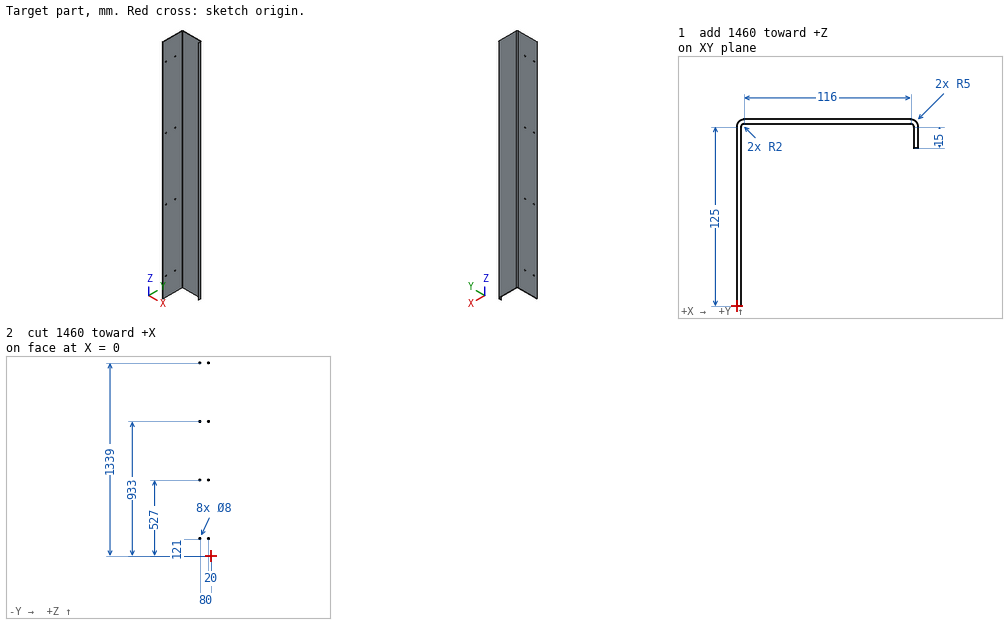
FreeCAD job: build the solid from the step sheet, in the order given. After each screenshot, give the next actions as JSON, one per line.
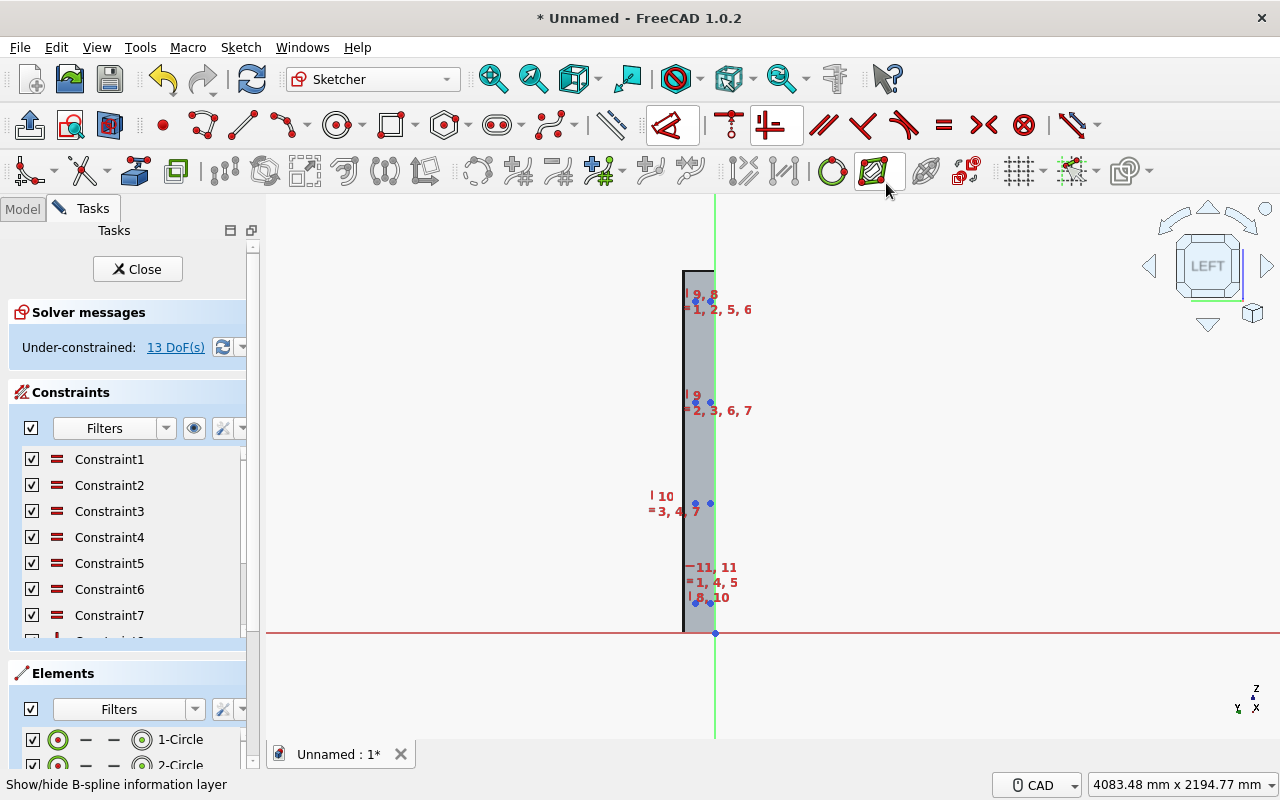
{"action": "left_click", "coordinate": [710, 604]}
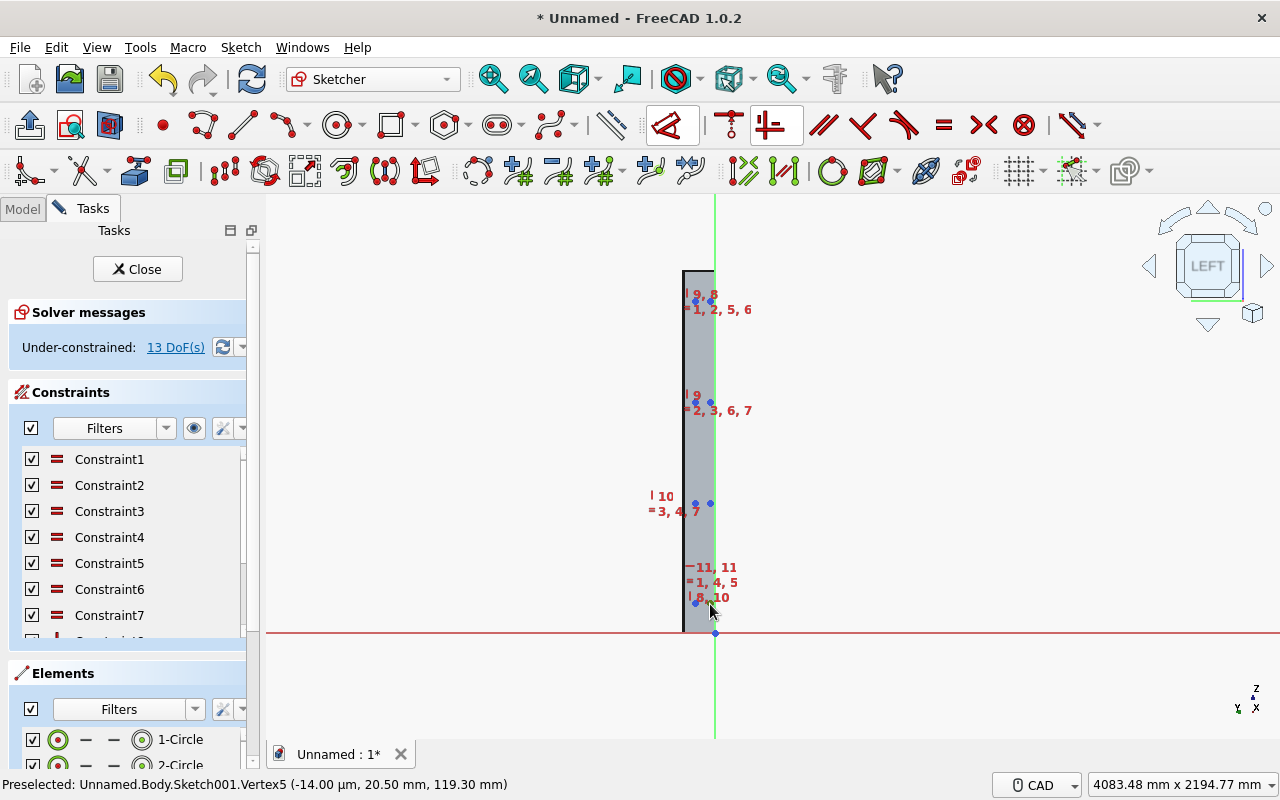
{"action": "left_click", "coordinate": [710, 301]}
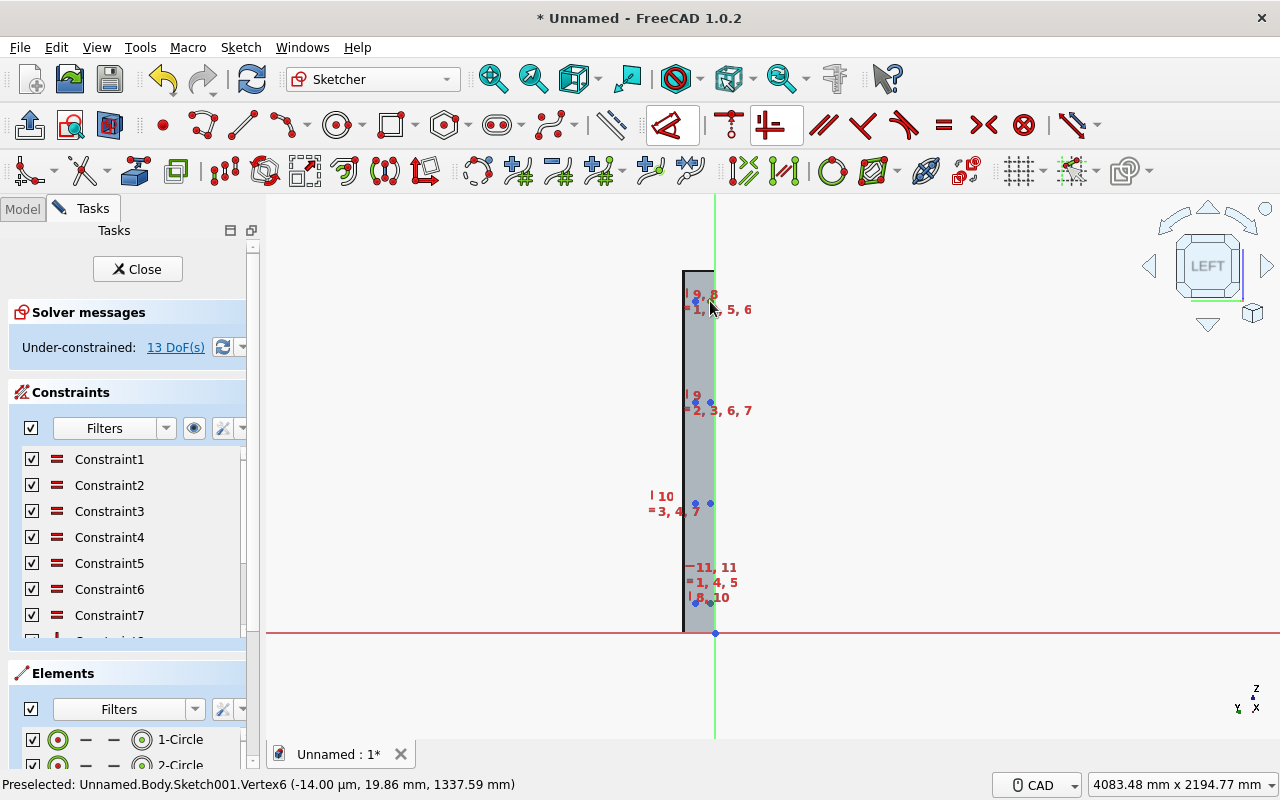
{"action": "left_click", "coordinate": [798, 126]}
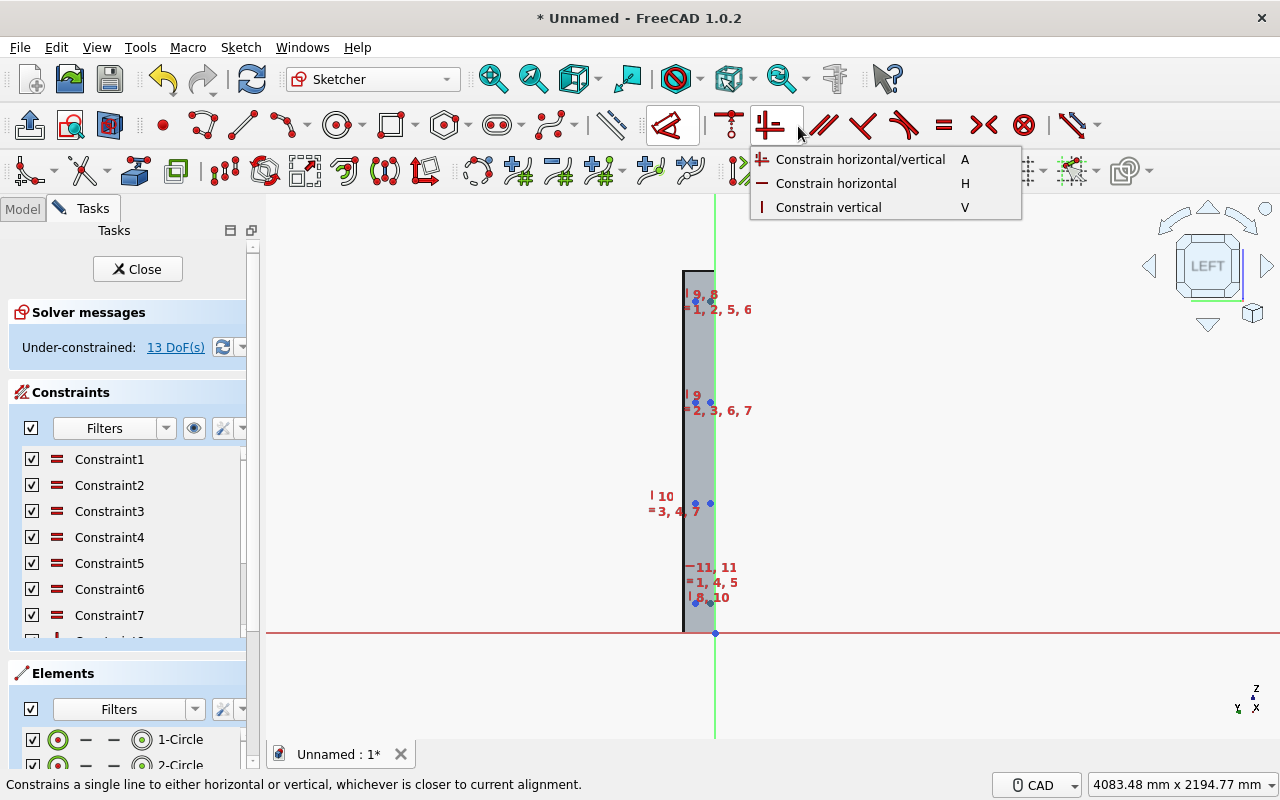
{"action": "left_click", "coordinate": [886, 207]}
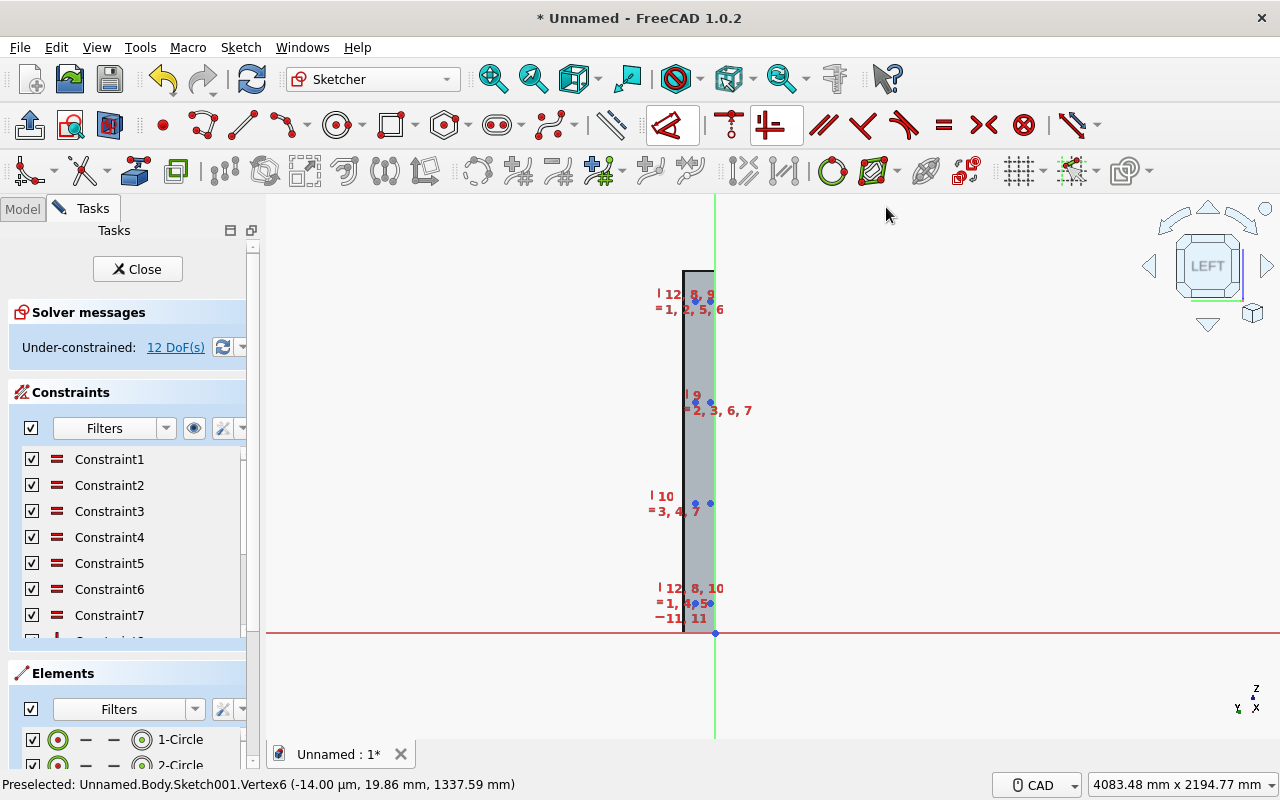
{"action": "scroll", "coordinate": [695, 302], "scroll_direction": "up", "scroll_amount": 4}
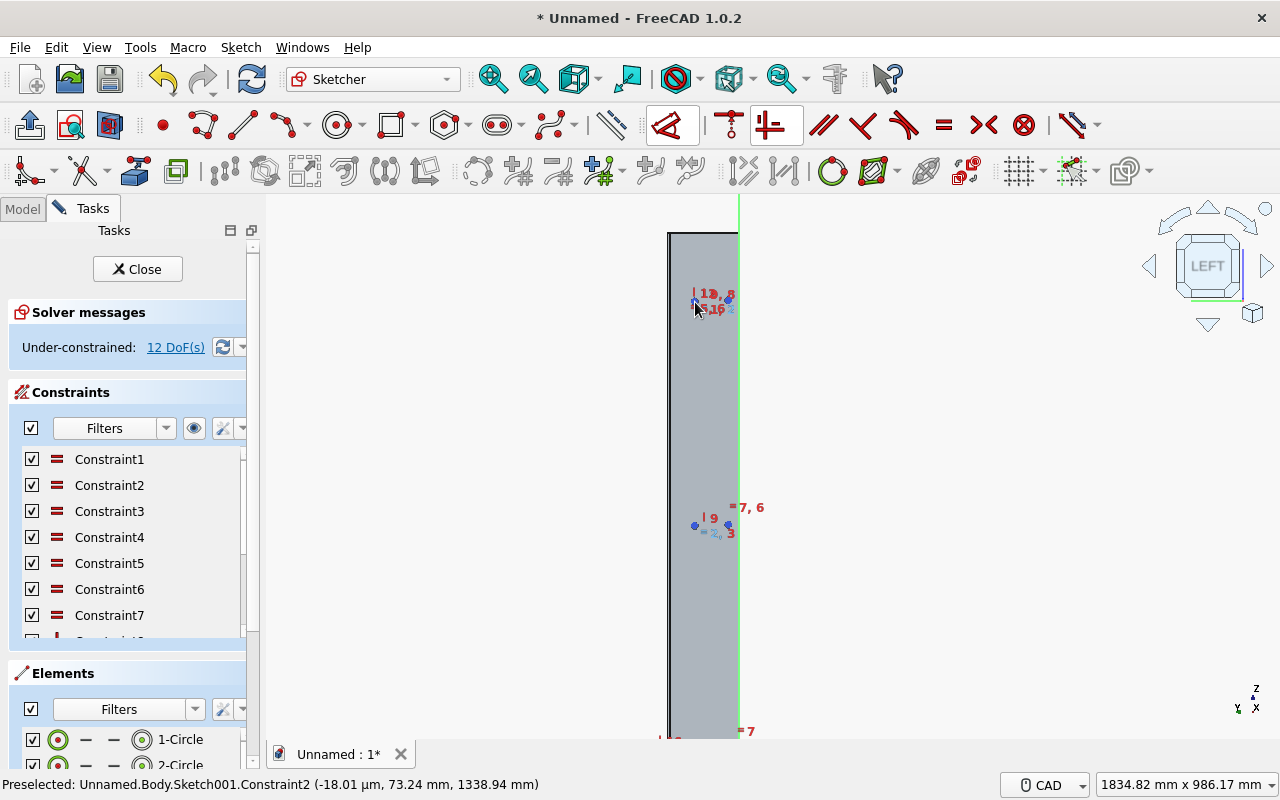
{"action": "scroll", "coordinate": [695, 302], "scroll_direction": "up", "scroll_amount": 4}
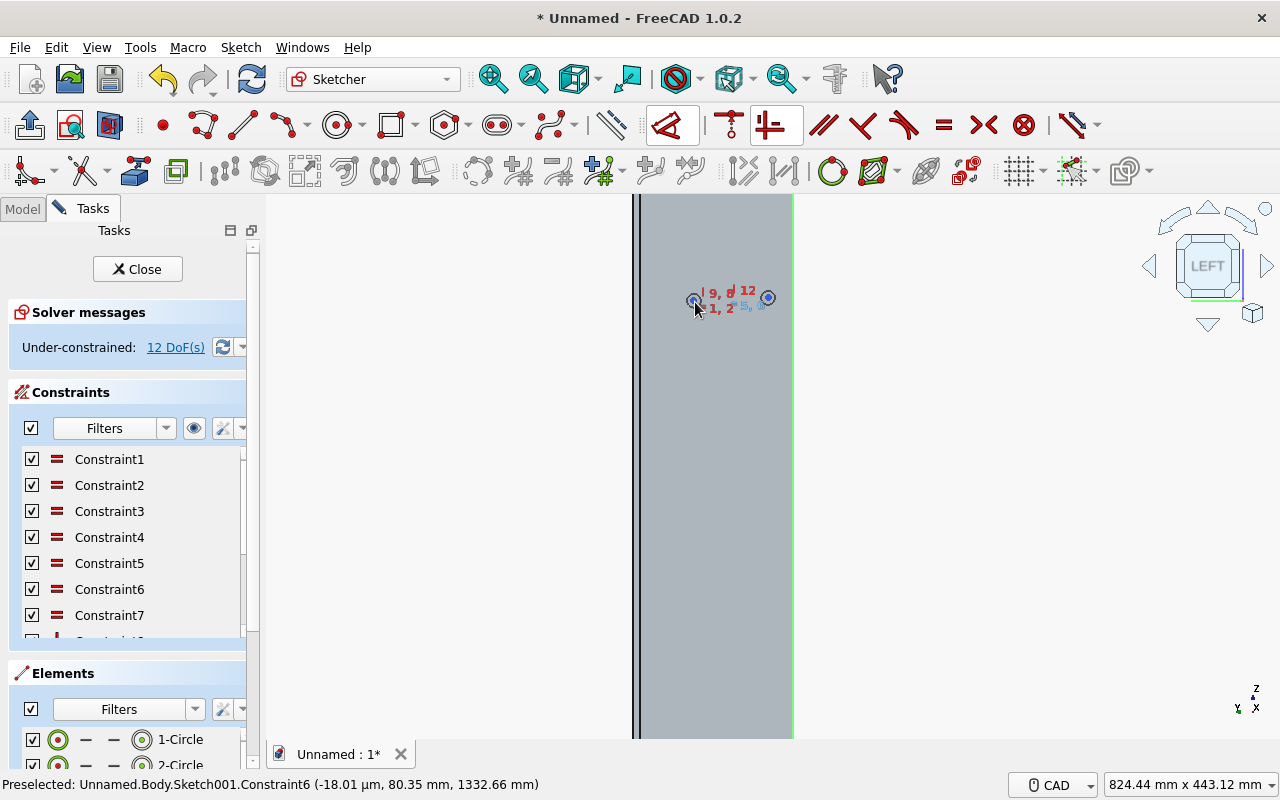
{"action": "left_click", "coordinate": [694, 301]}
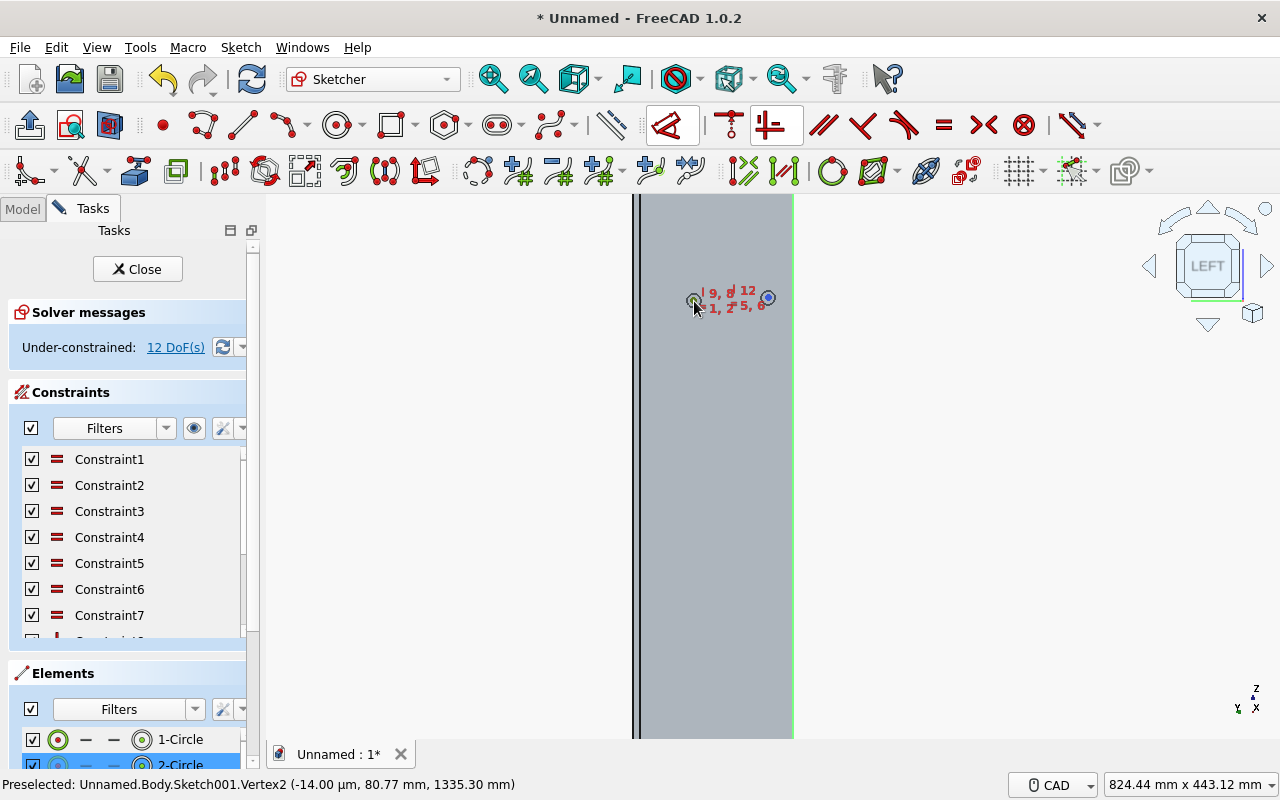
{"action": "scroll", "coordinate": [695, 302], "scroll_direction": "down", "scroll_amount": 8}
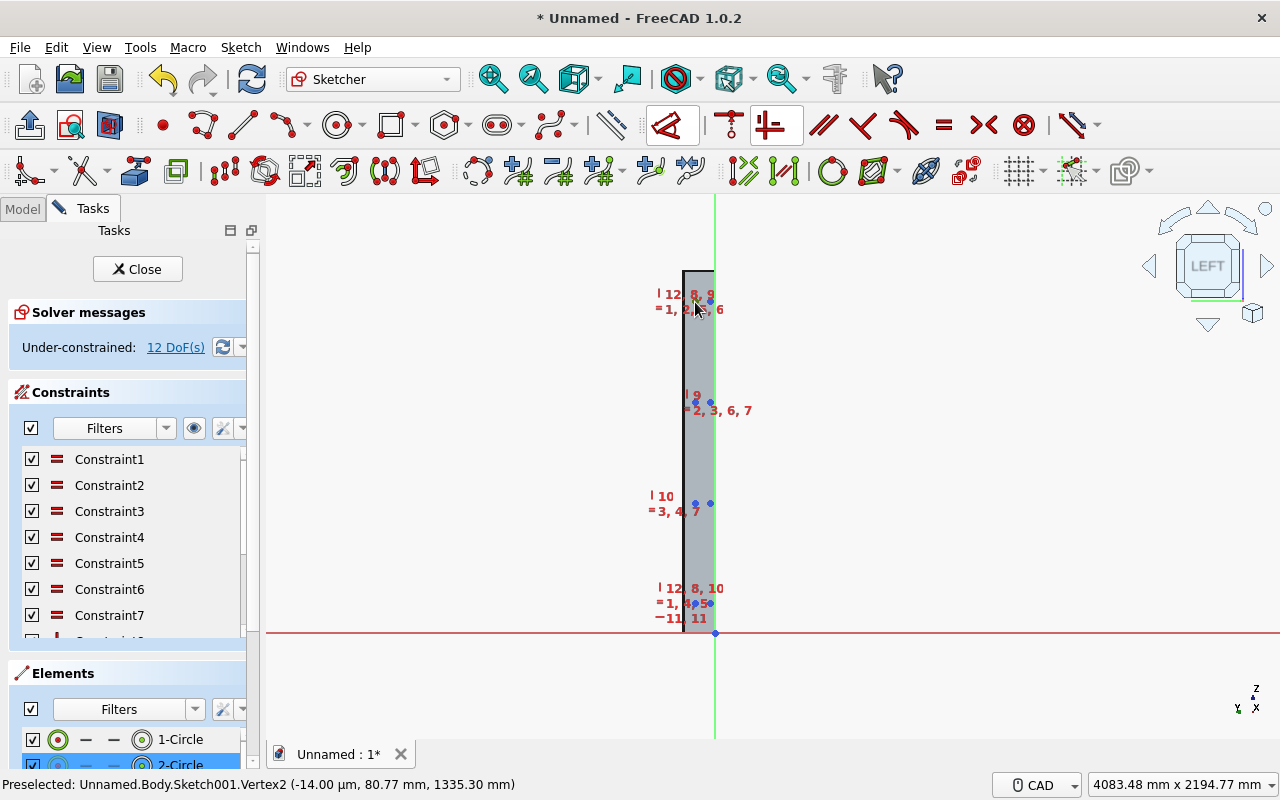
{"action": "scroll", "coordinate": [710, 301], "scroll_direction": "up", "scroll_amount": 4}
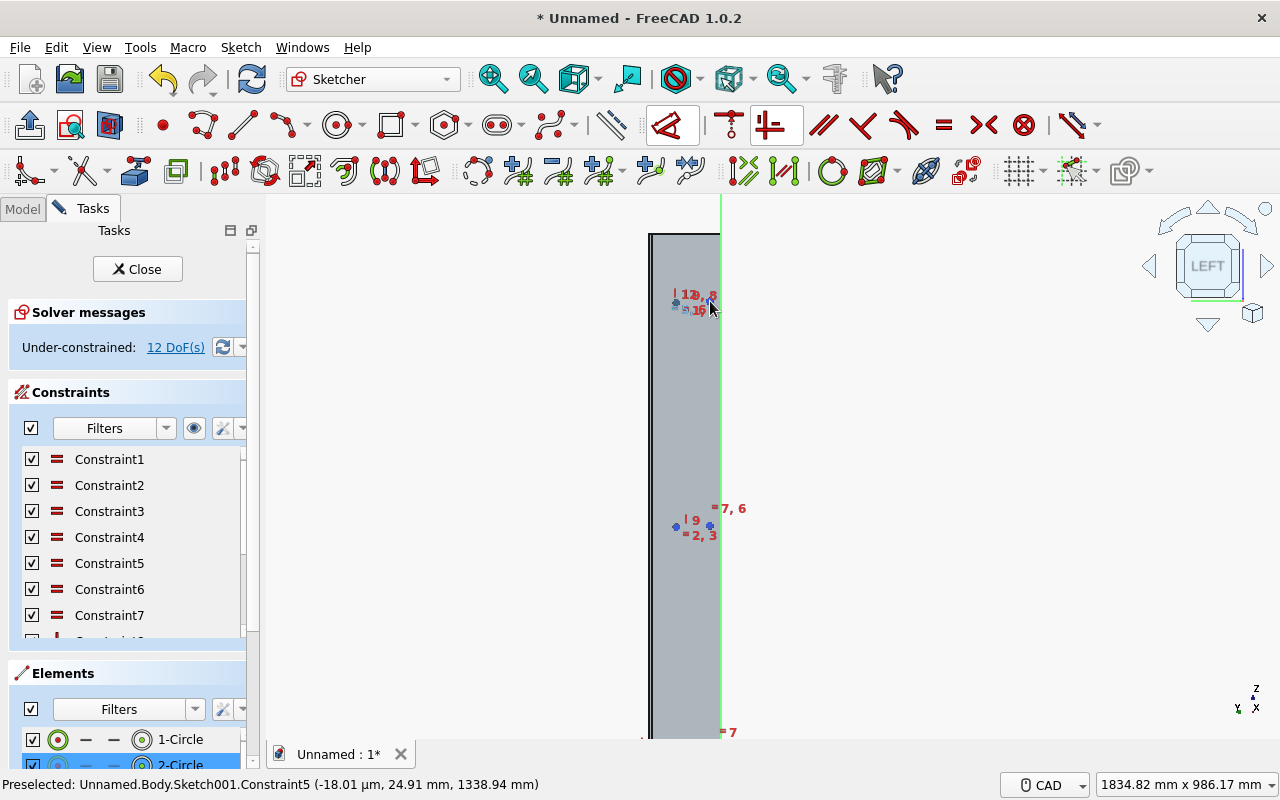
{"action": "left_click", "coordinate": [710, 302]}